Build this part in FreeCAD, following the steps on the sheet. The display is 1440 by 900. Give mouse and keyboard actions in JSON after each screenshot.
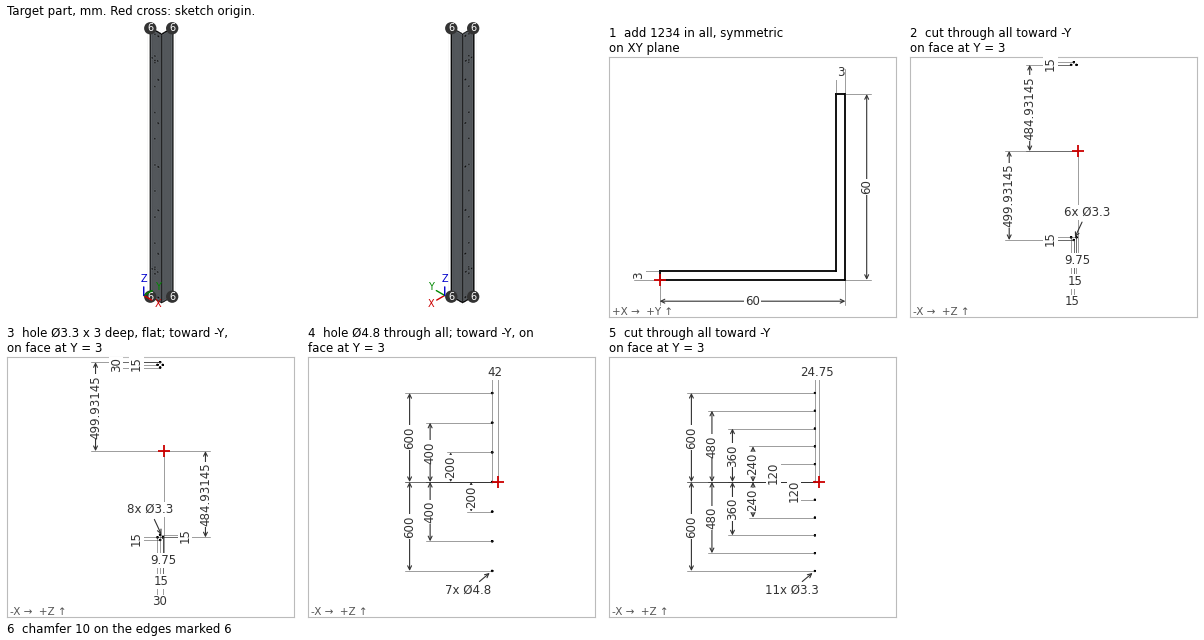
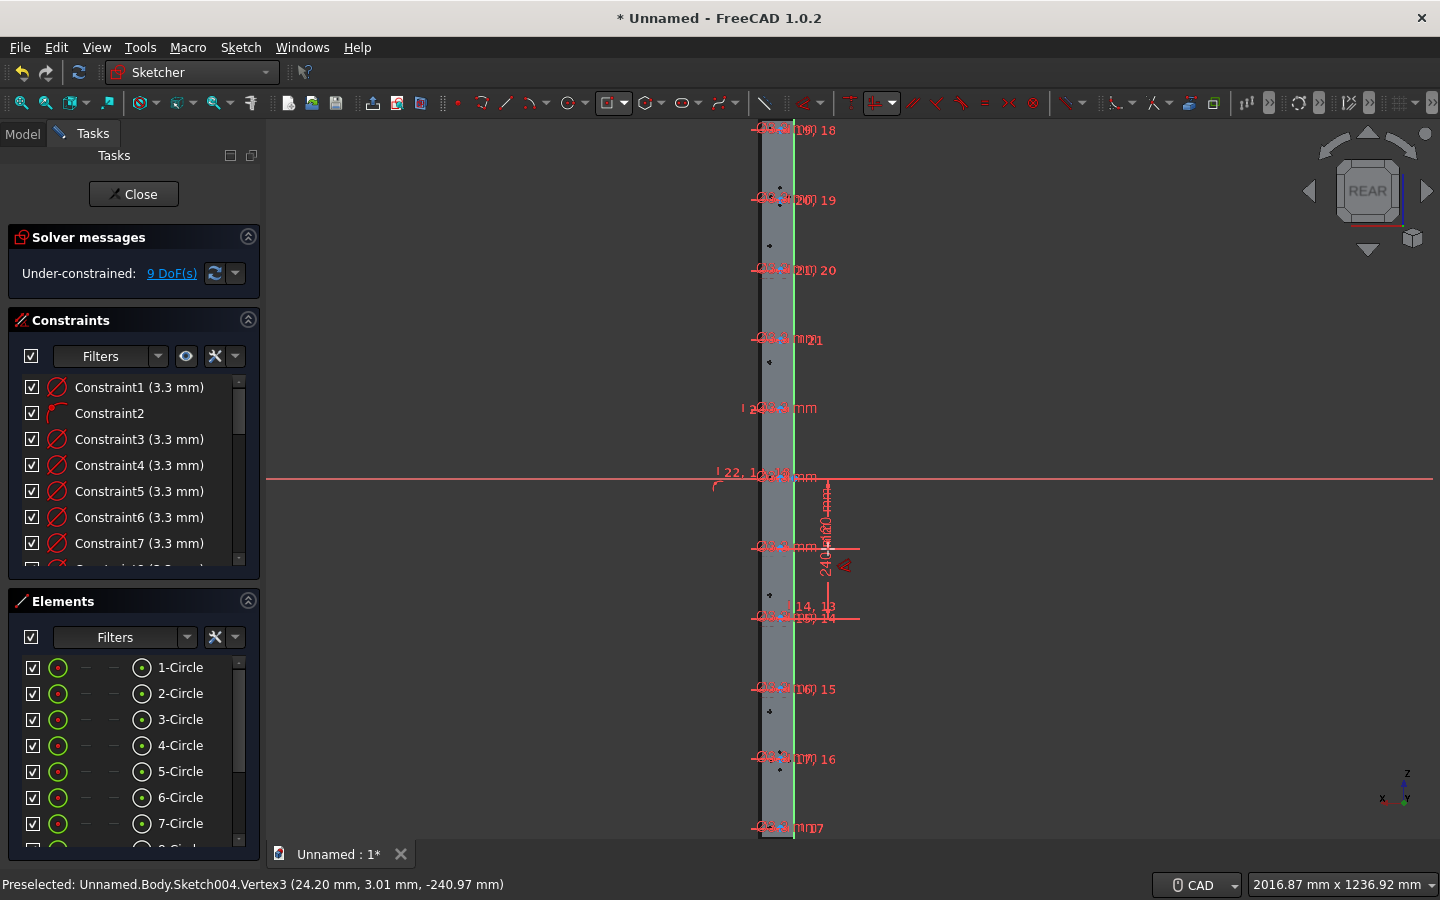
{"action": "left_click", "coordinate": [780, 690]}
{"action": "left_click", "coordinate": [828, 584]}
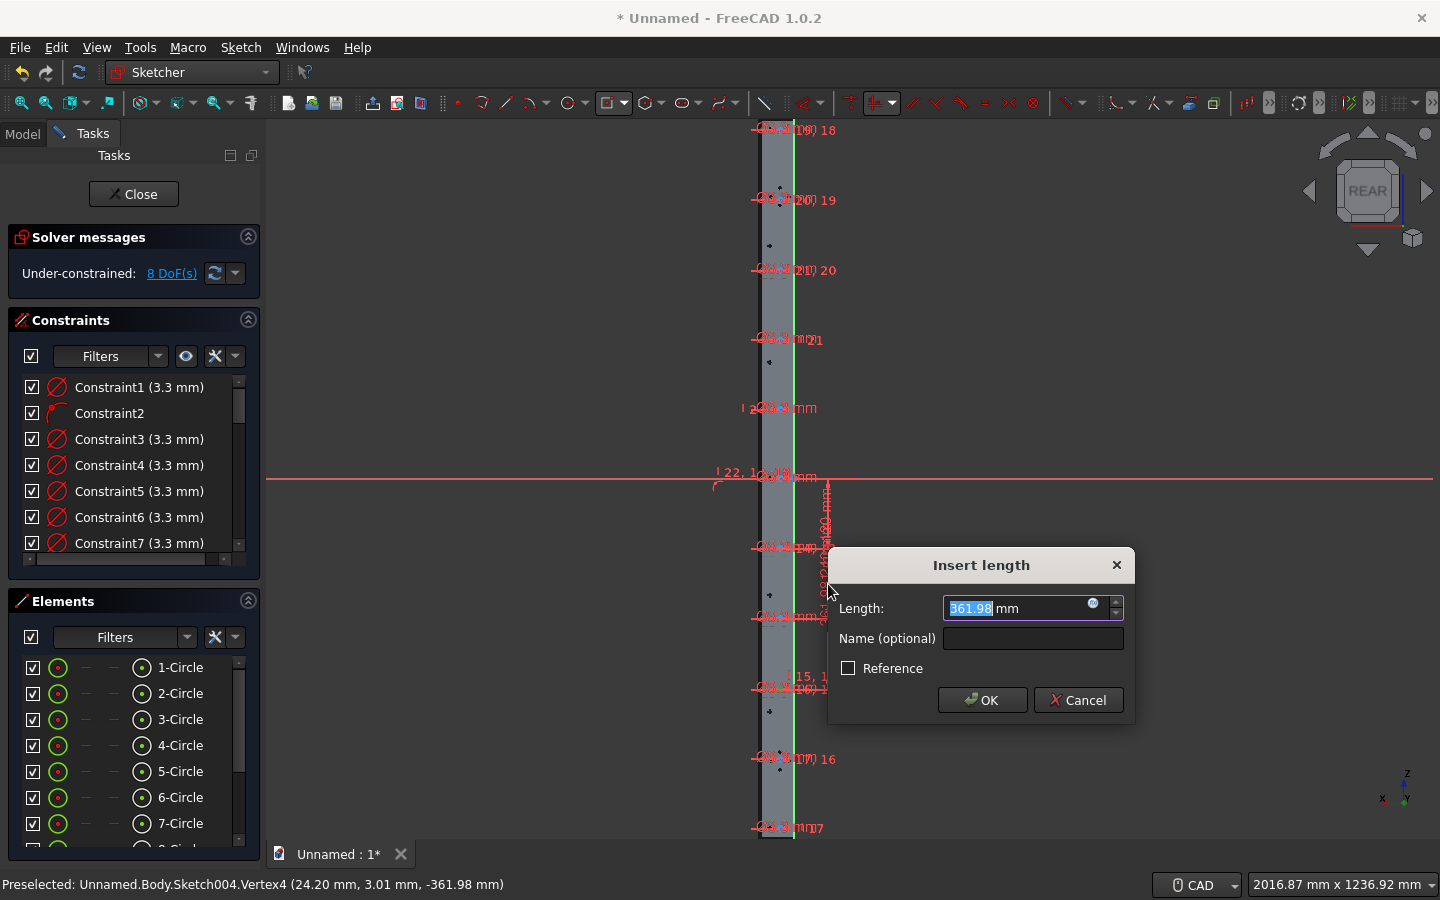
{"action": "type", "text": "360"}
{"action": "key", "text": "Return"}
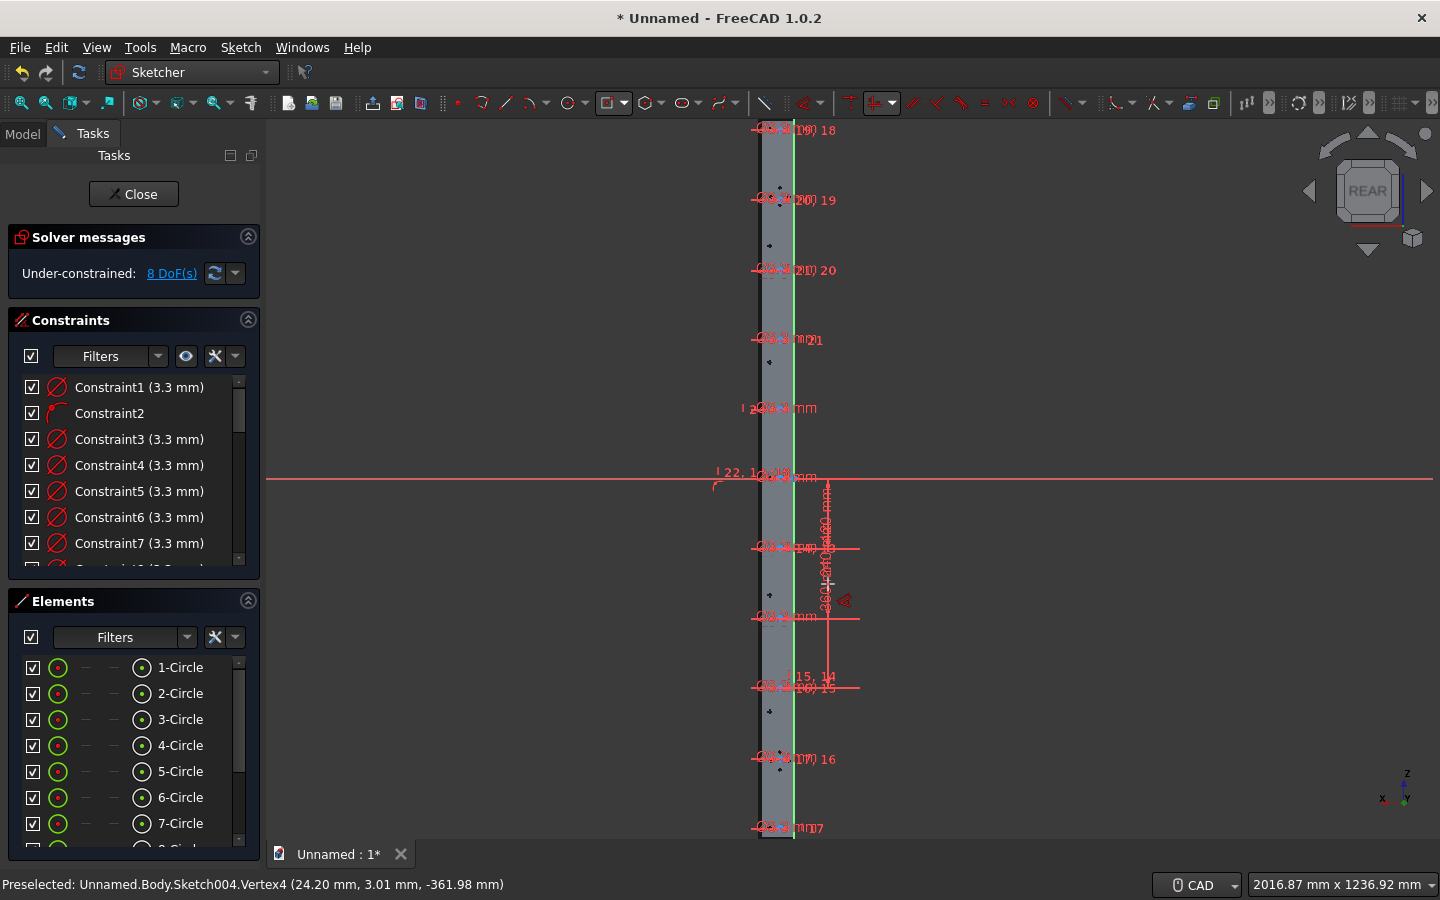
{"action": "left_click", "coordinate": [780, 759]}
{"action": "left_click", "coordinate": [828, 619]}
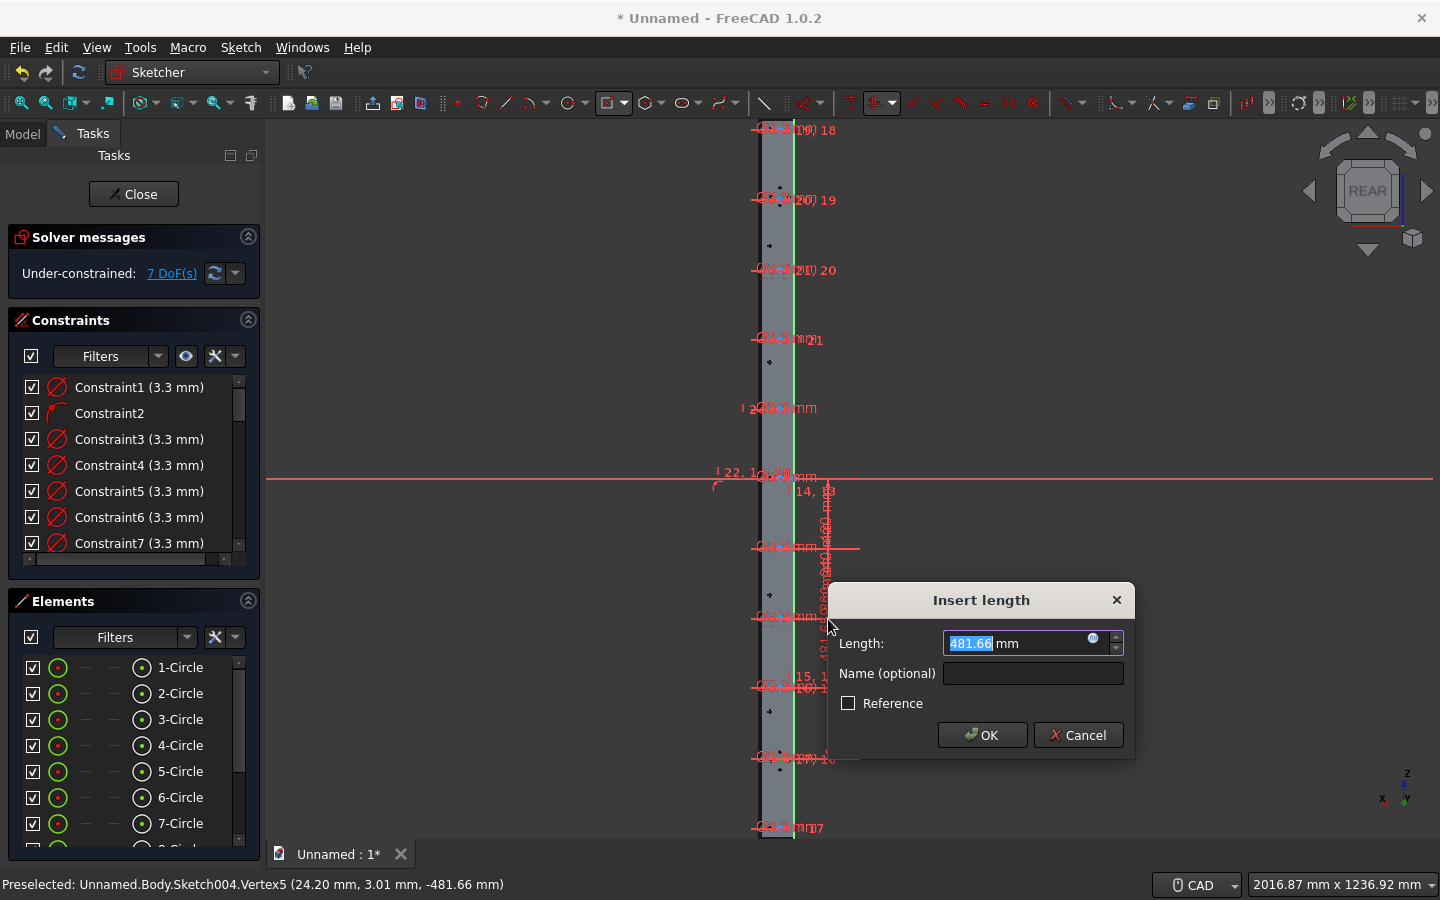
{"action": "type", "text": "480"}
{"action": "key", "text": "Return"}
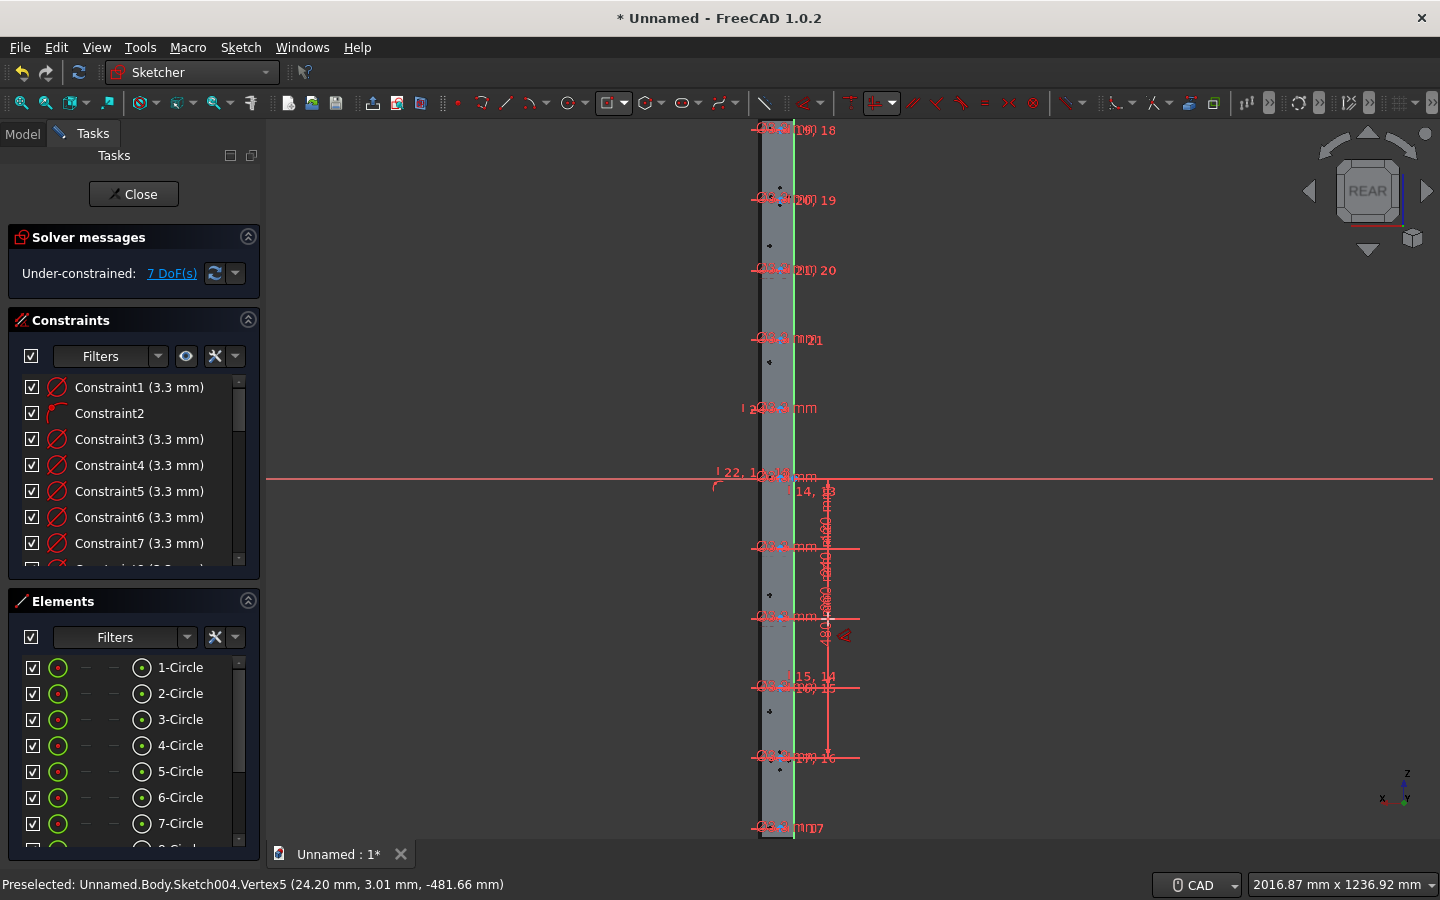
{"action": "scroll", "coordinate": [780, 479], "scroll_direction": "down", "scroll_amount": 2}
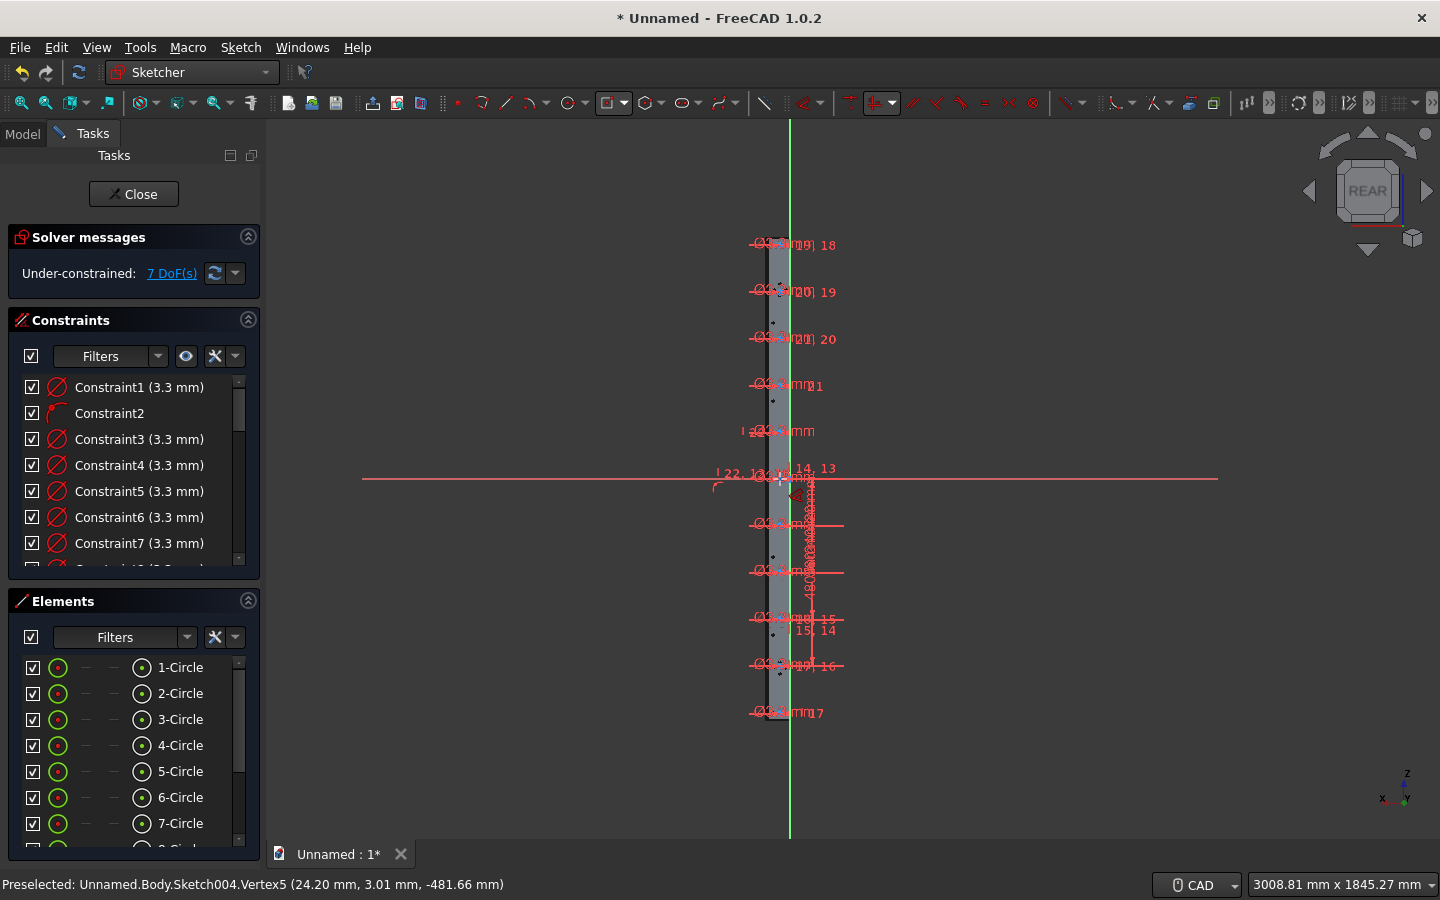
{"action": "left_click", "coordinate": [780, 714]}
{"action": "left_click", "coordinate": [824, 596]}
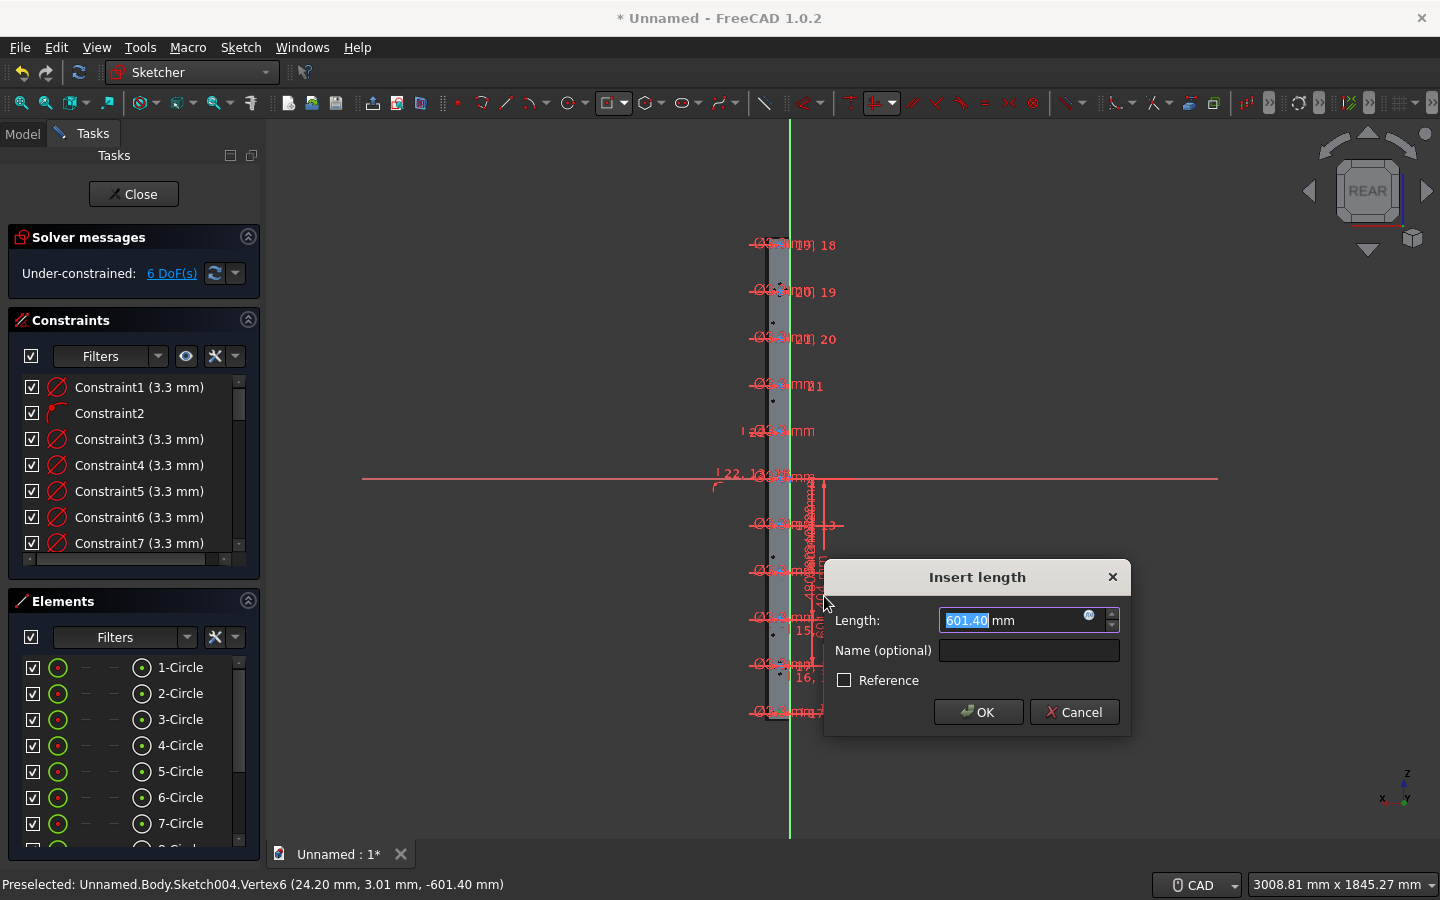
{"action": "type", "text": "600"}
{"action": "key", "text": "Return"}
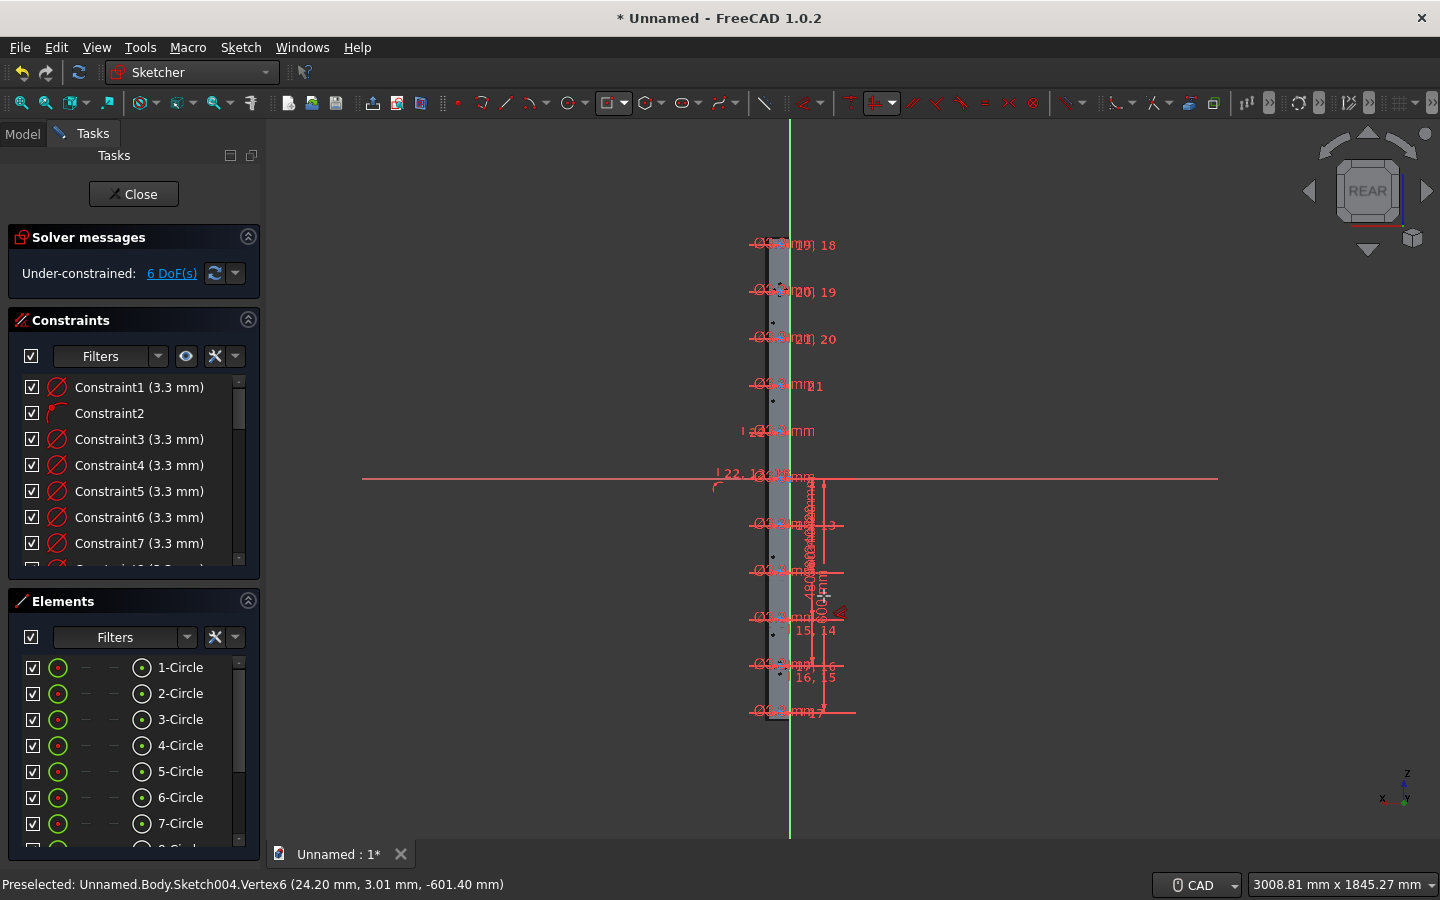
{"action": "left_click", "coordinate": [780, 245]}
{"action": "left_click", "coordinate": [824, 362]}